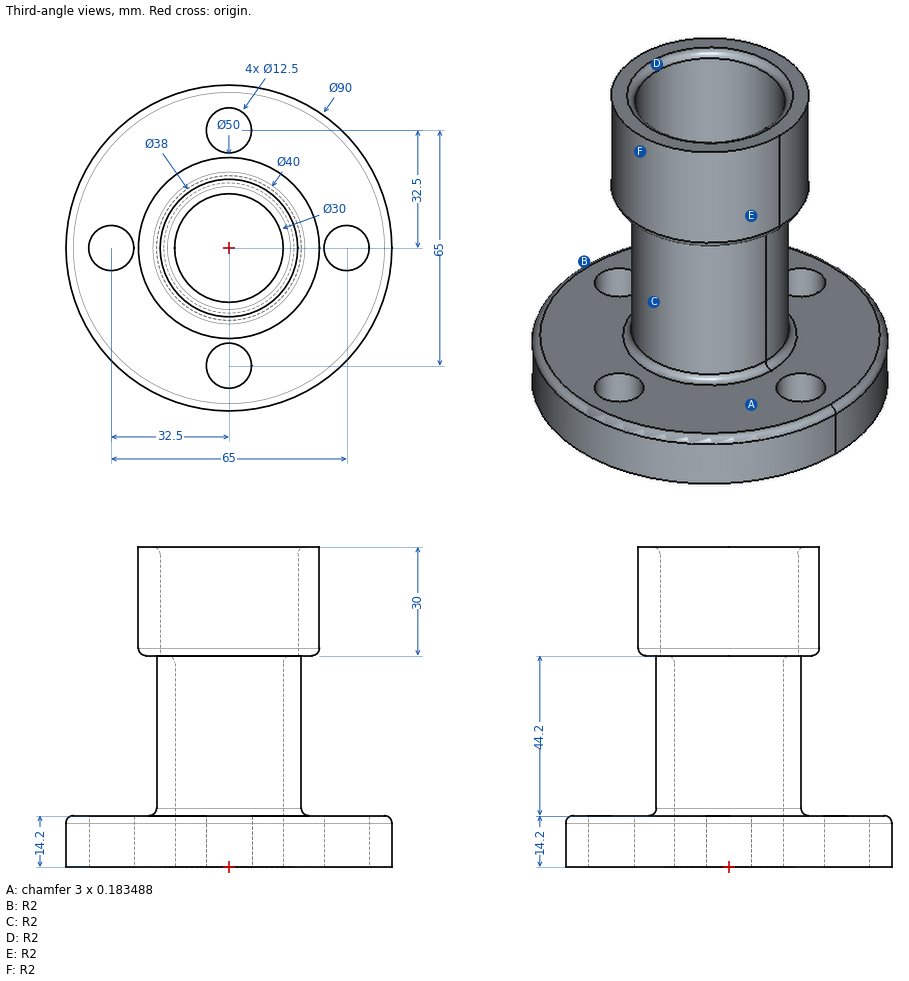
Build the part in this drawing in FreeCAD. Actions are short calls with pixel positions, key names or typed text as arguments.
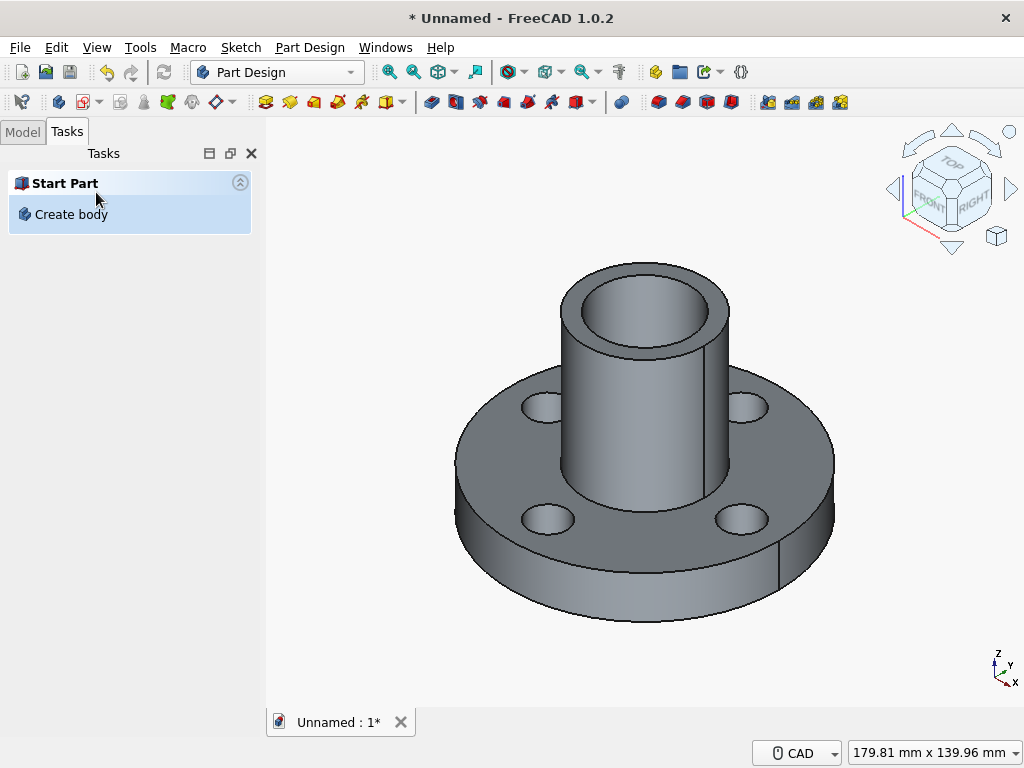
click(577, 291)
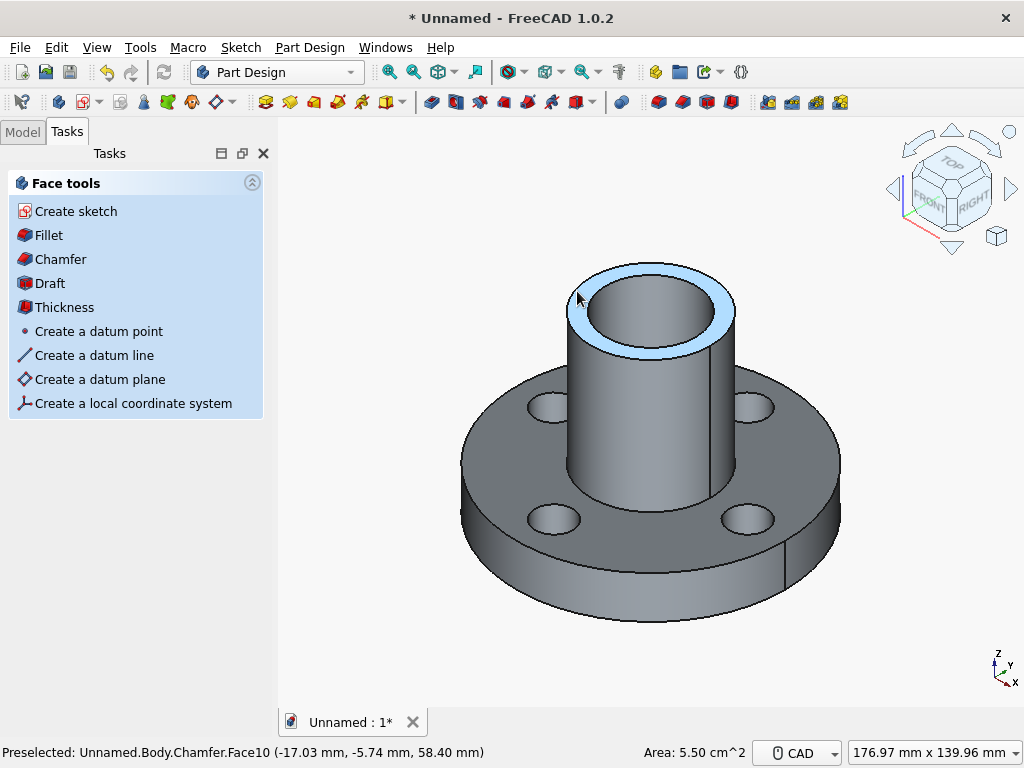
click(84, 102)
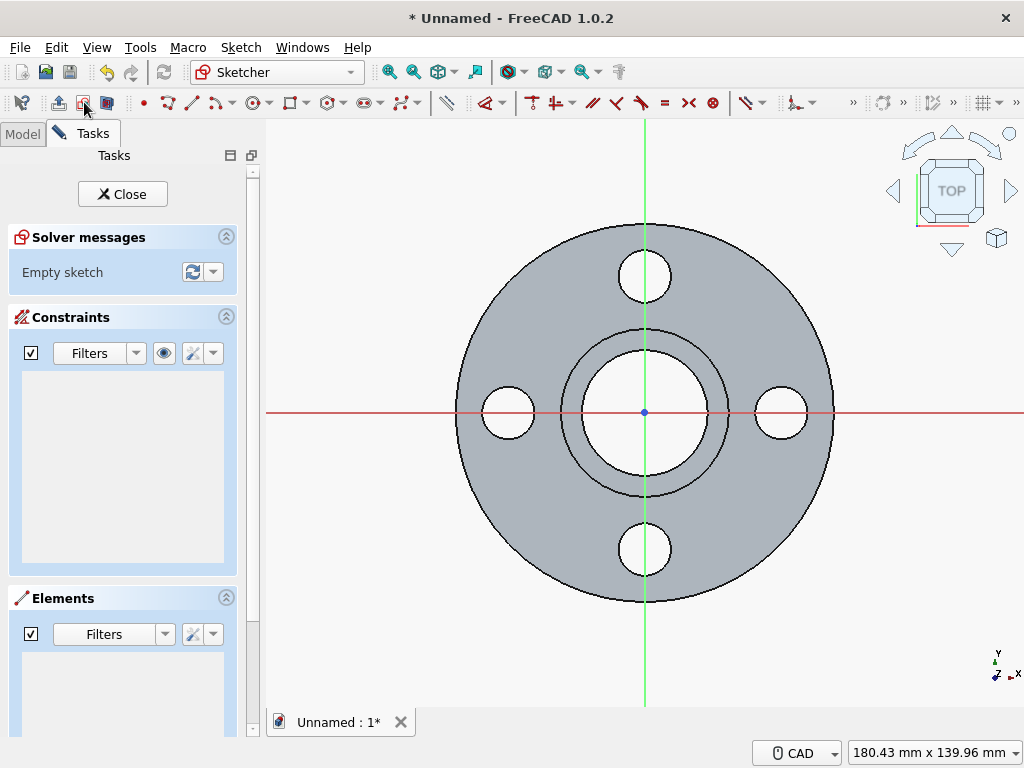
scroll(728, 413, up, 3)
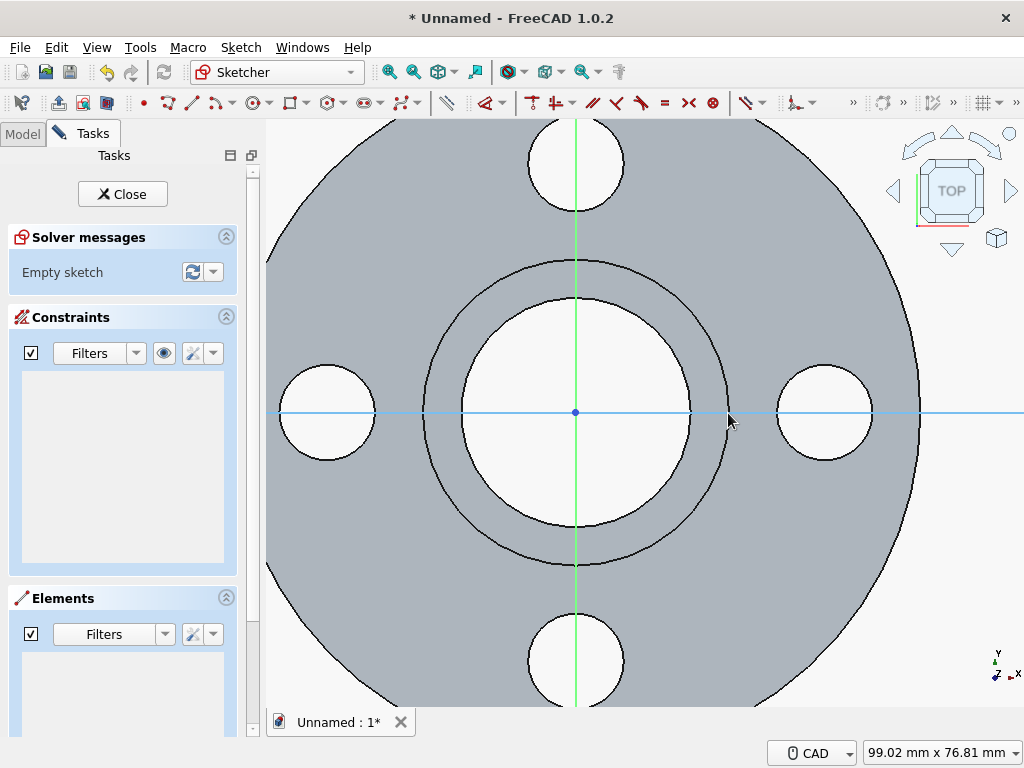
key(g)
key(c)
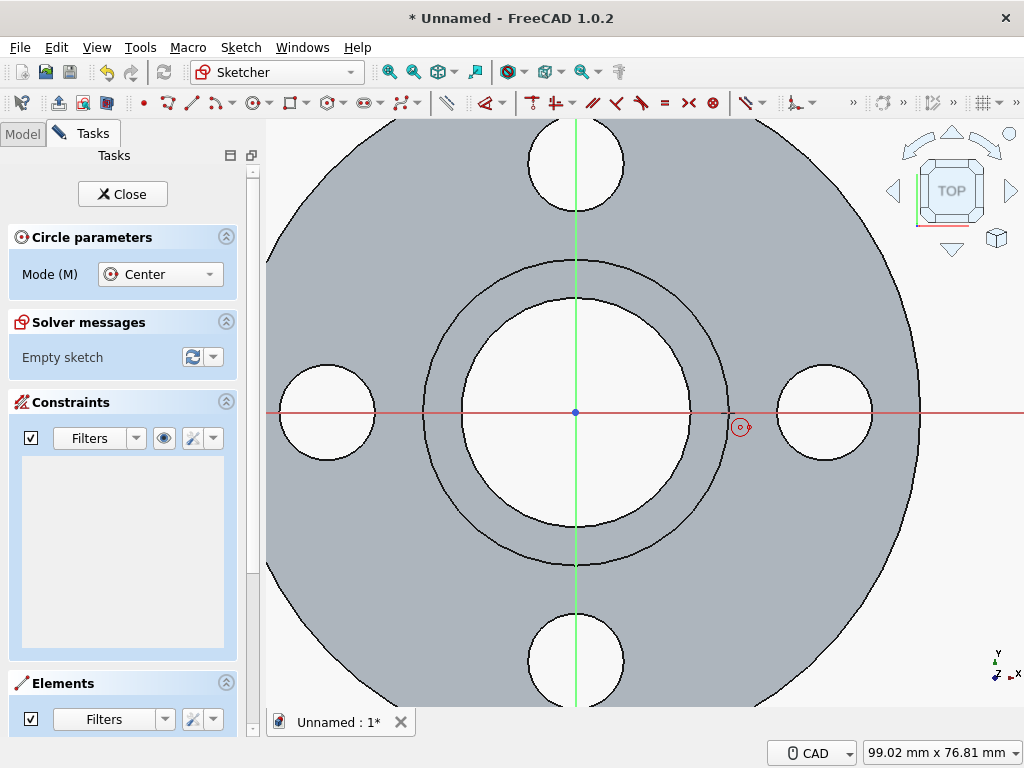
click(576, 413)
move(711, 277)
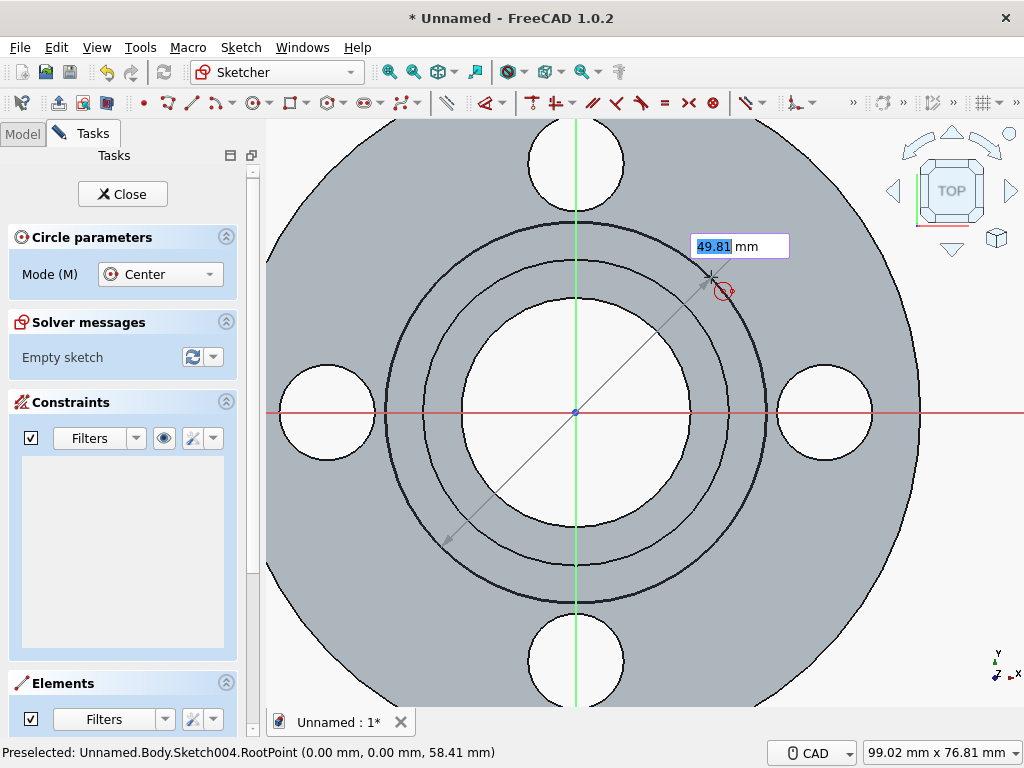
text(50)
key(Return)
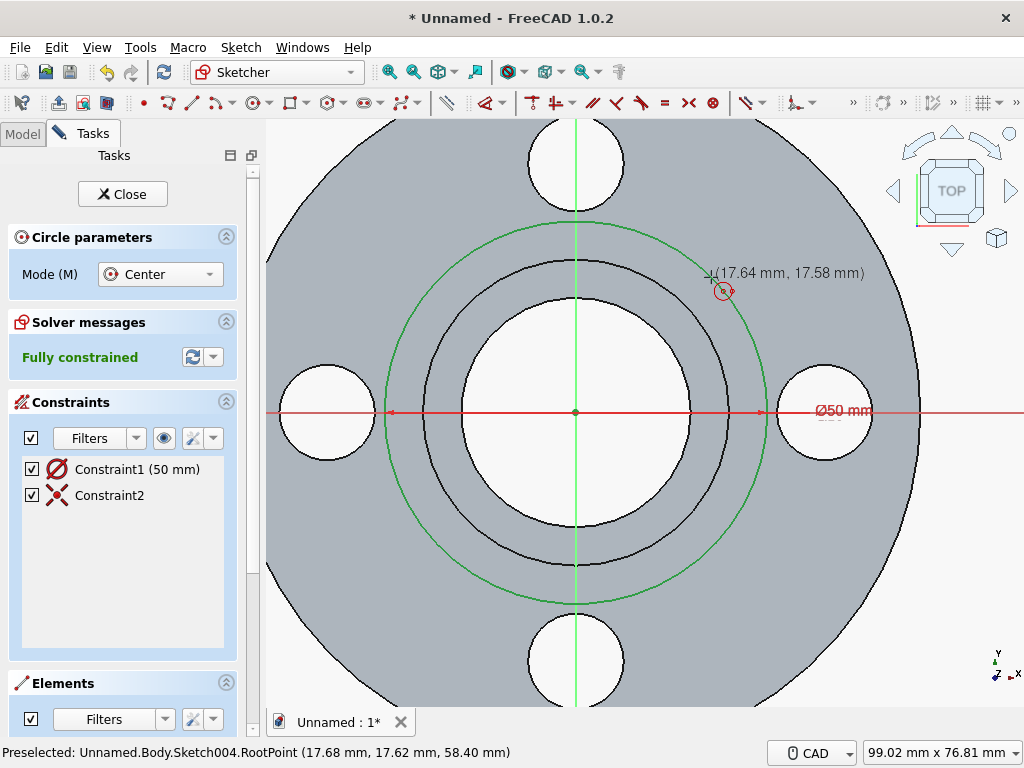
click(576, 413)
move(679, 310)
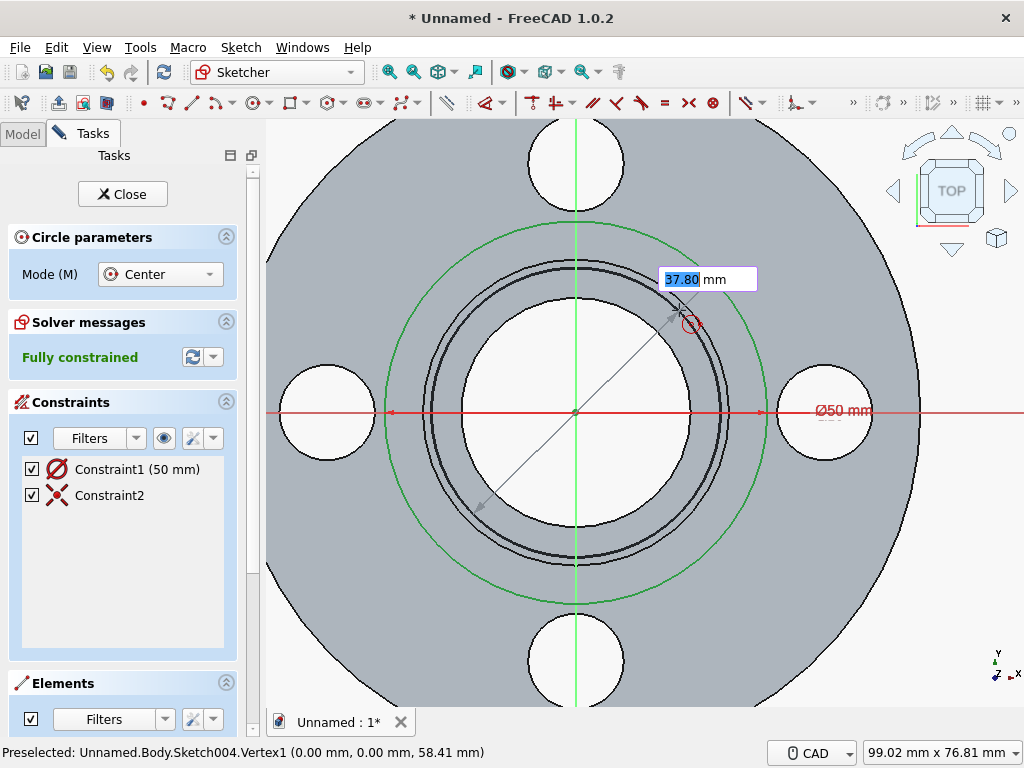
text(38)
key(Return)
key(Escape)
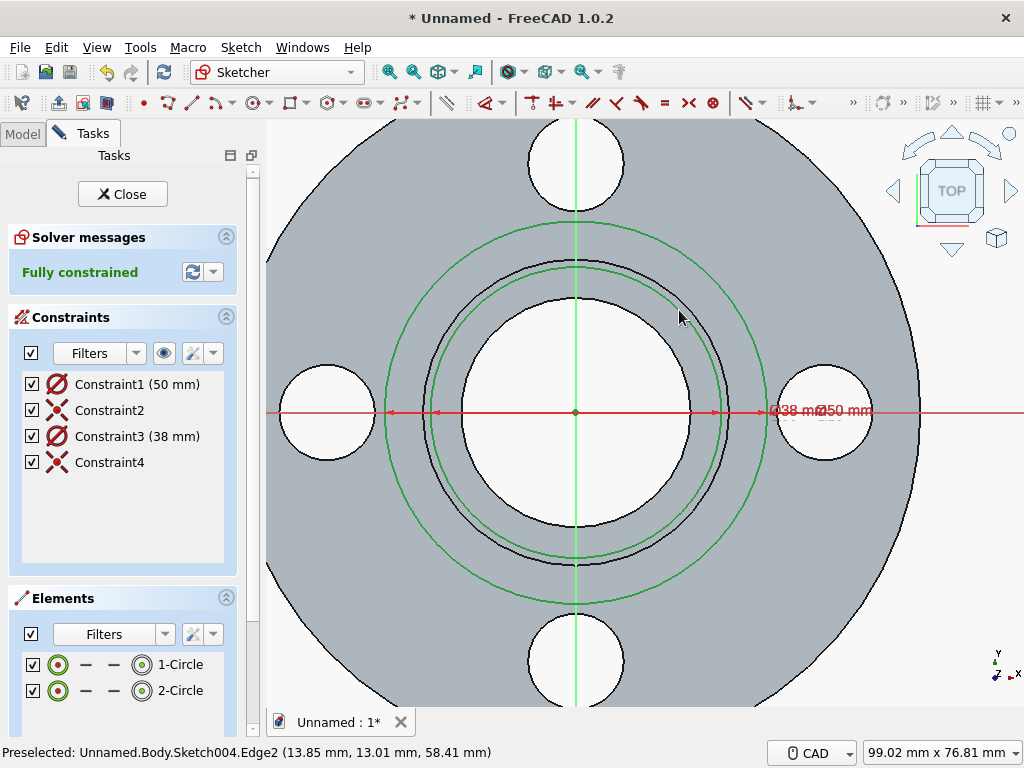
click(123, 194)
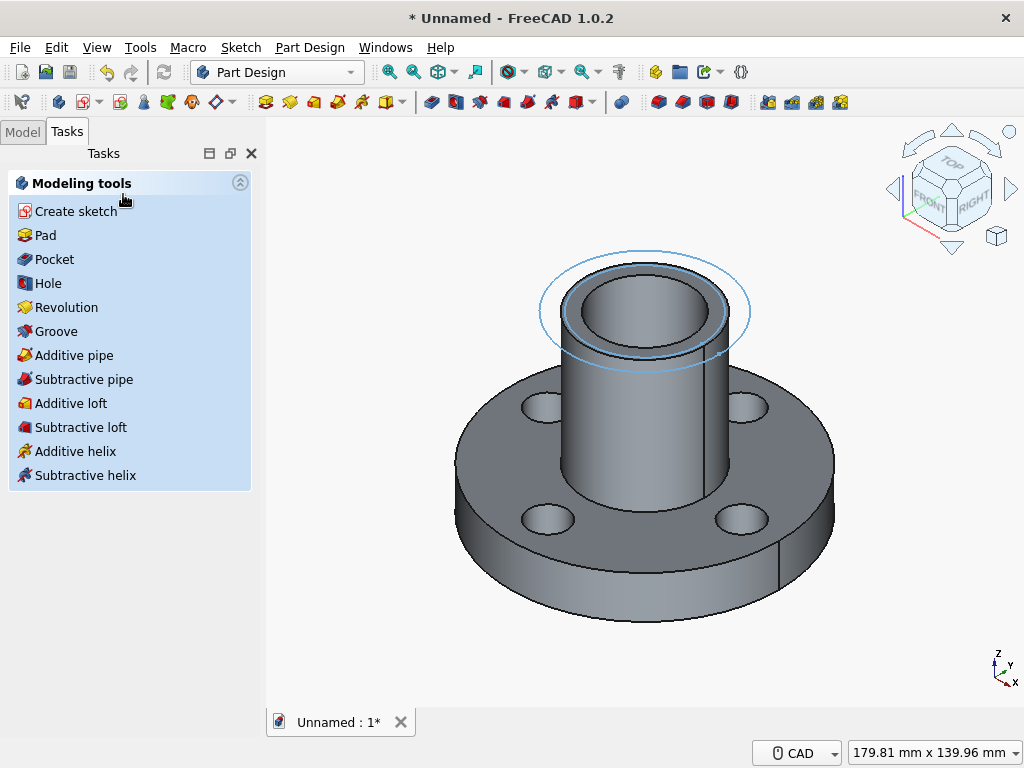
click(266, 102)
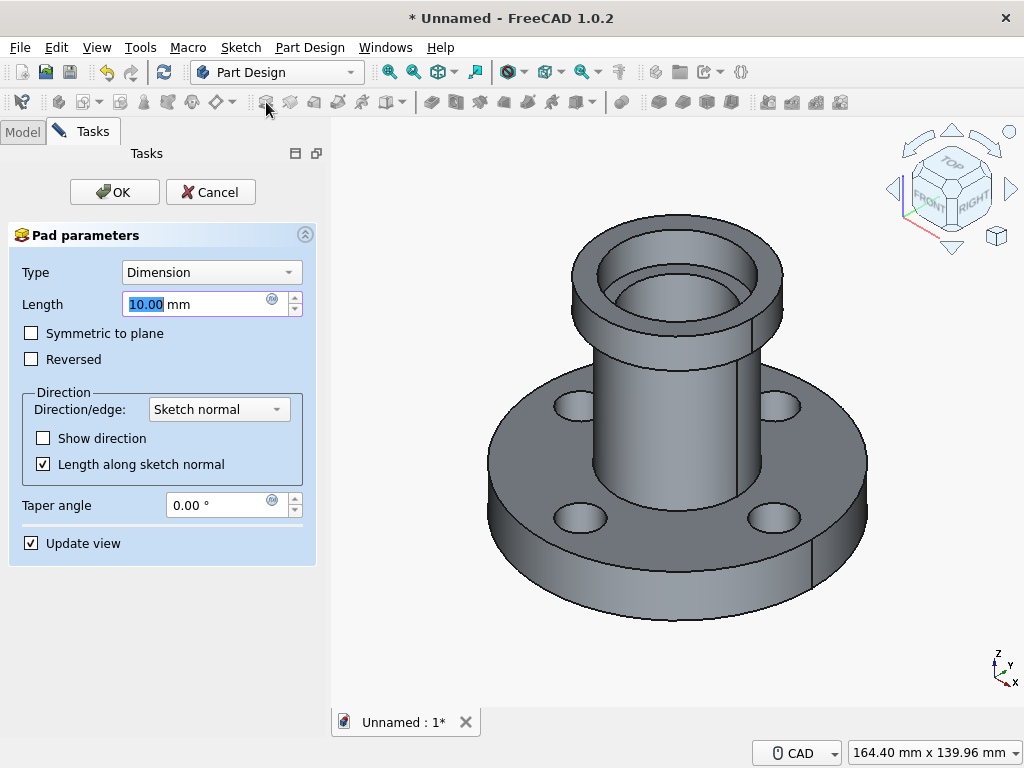
text(30)
key(Tab)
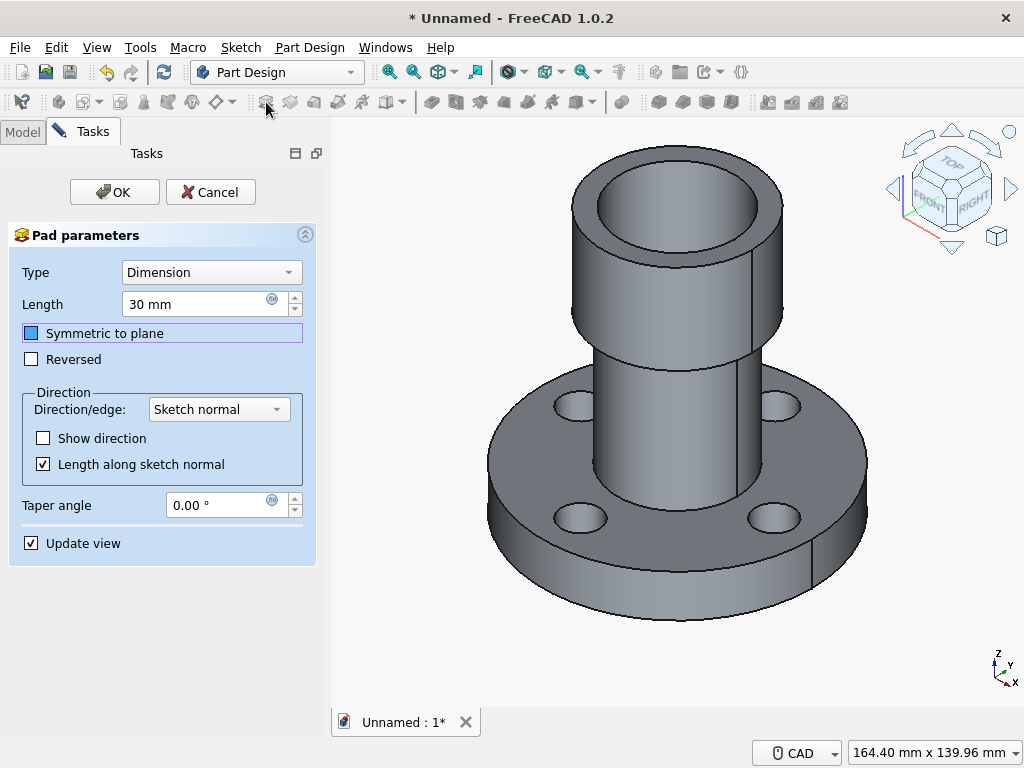
click(115, 192)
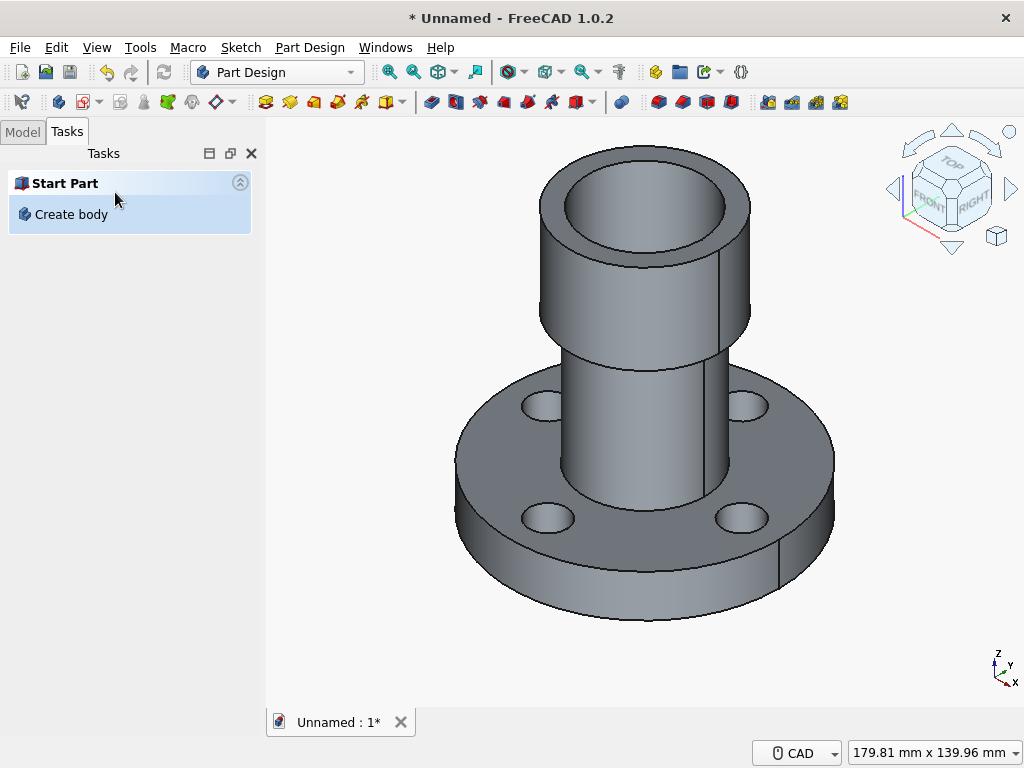
click(390, 72)